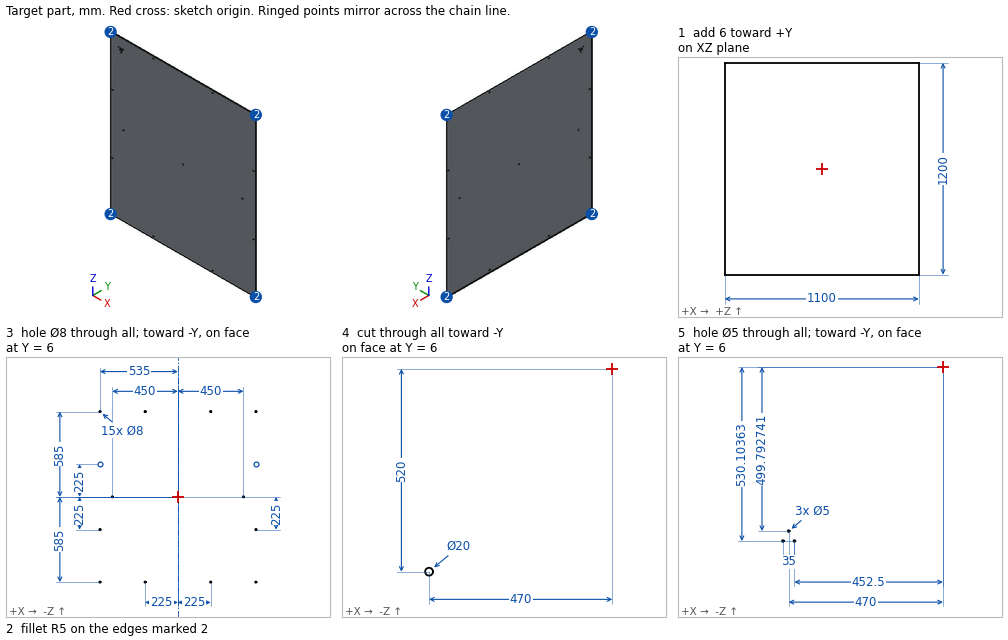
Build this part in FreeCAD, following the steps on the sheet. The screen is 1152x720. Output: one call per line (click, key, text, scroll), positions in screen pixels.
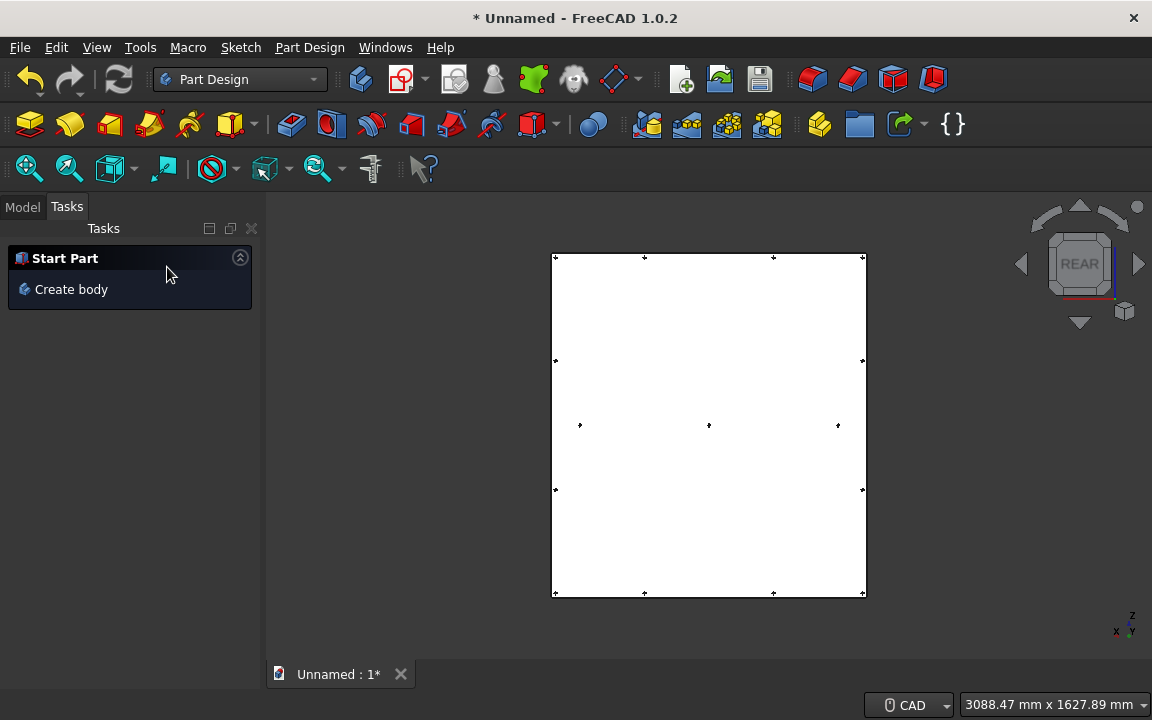
click(709, 523)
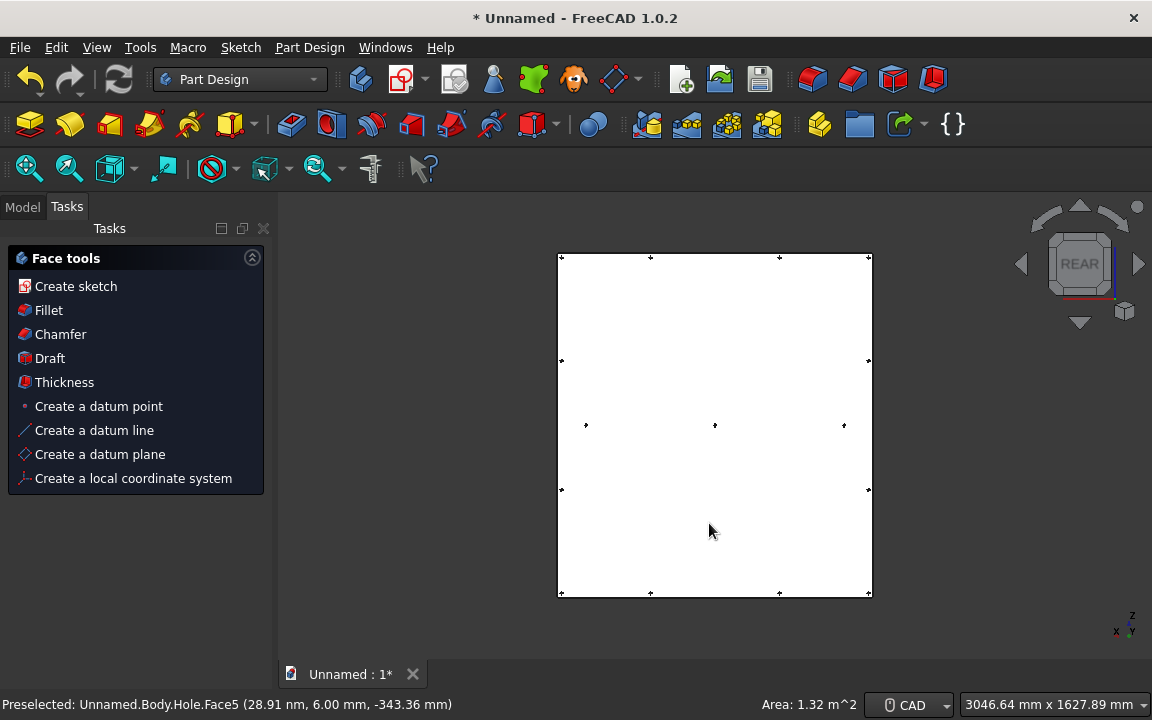
click(402, 80)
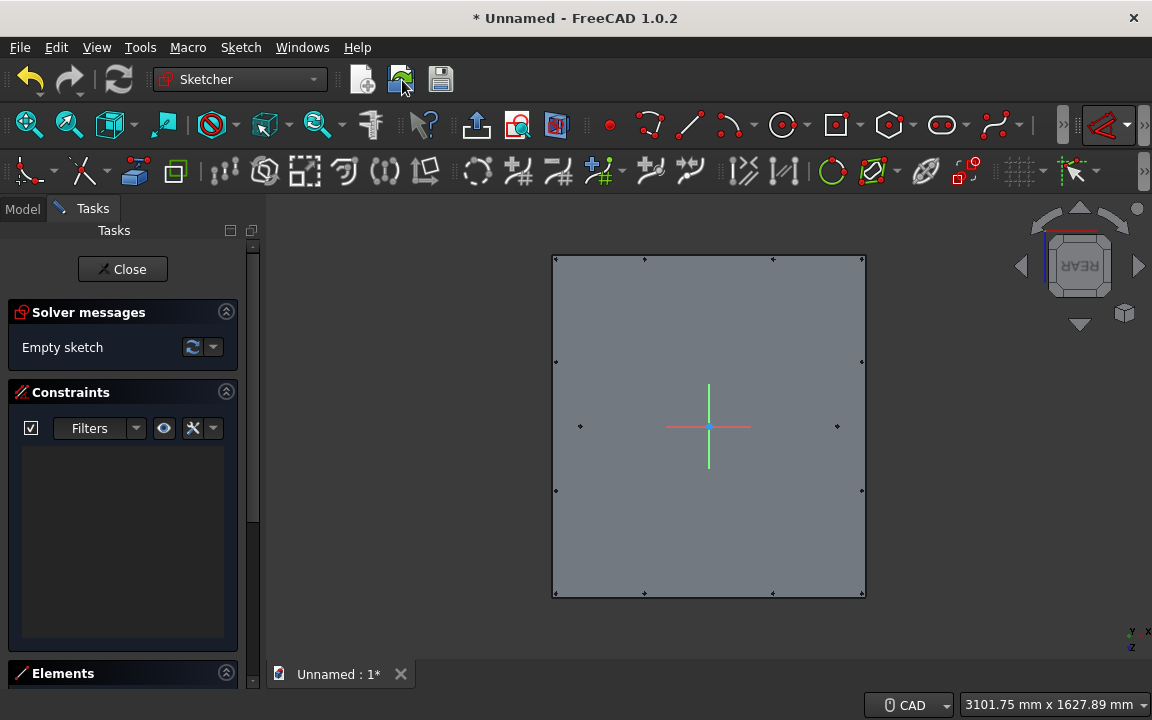
scroll(571, 583, up, 15)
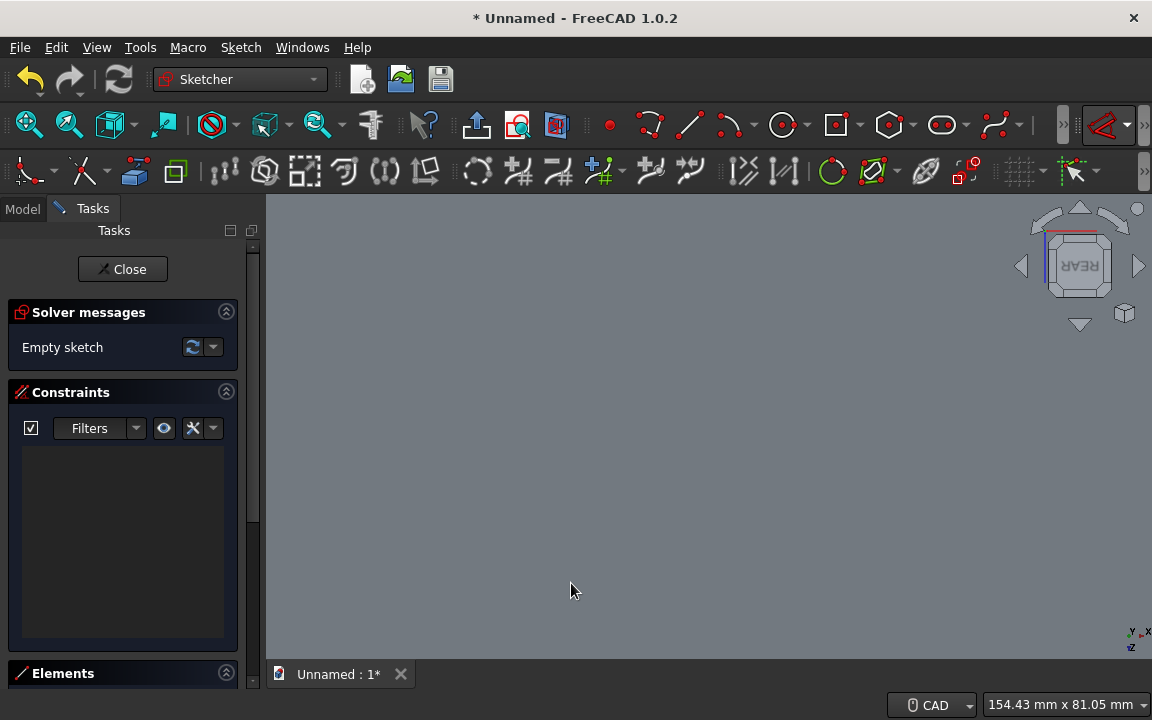
scroll(639, 396, up, 5)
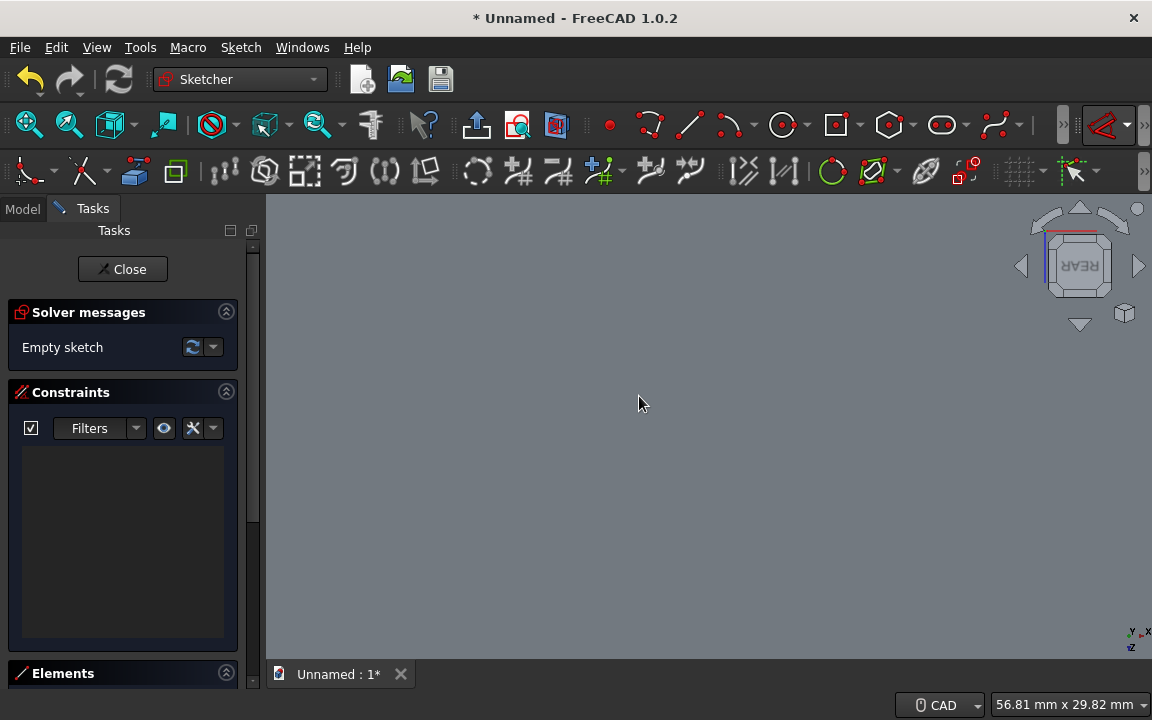
click(784, 126)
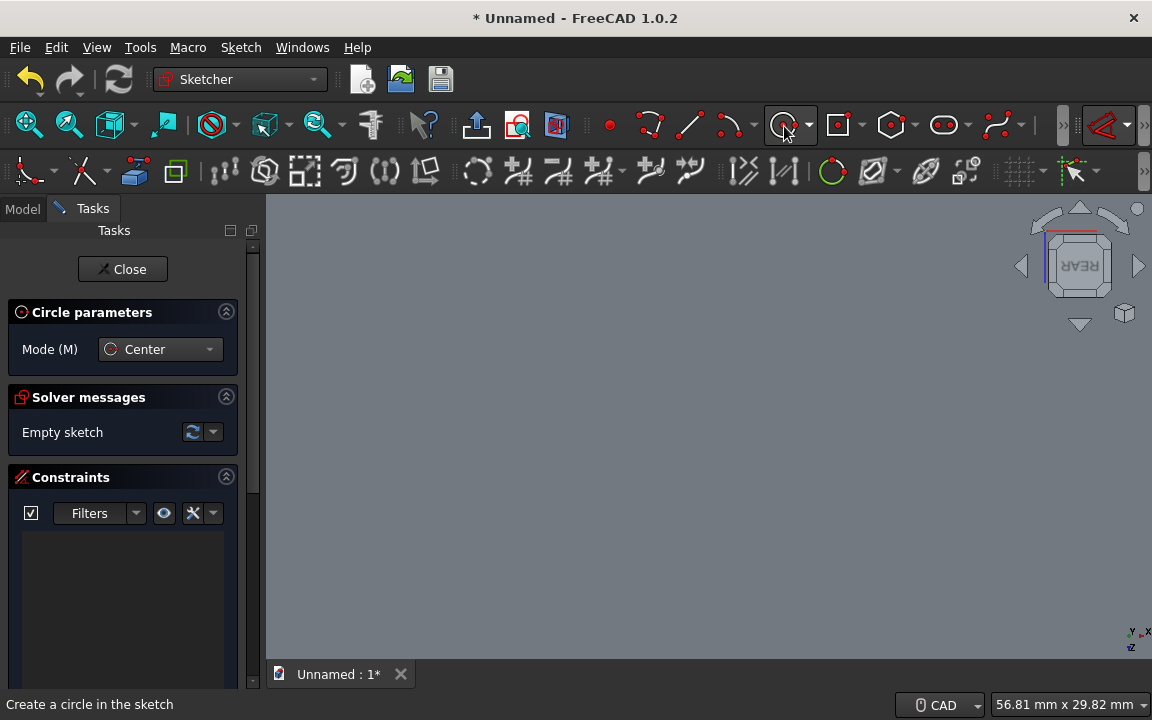
click(640, 425)
move(750, 315)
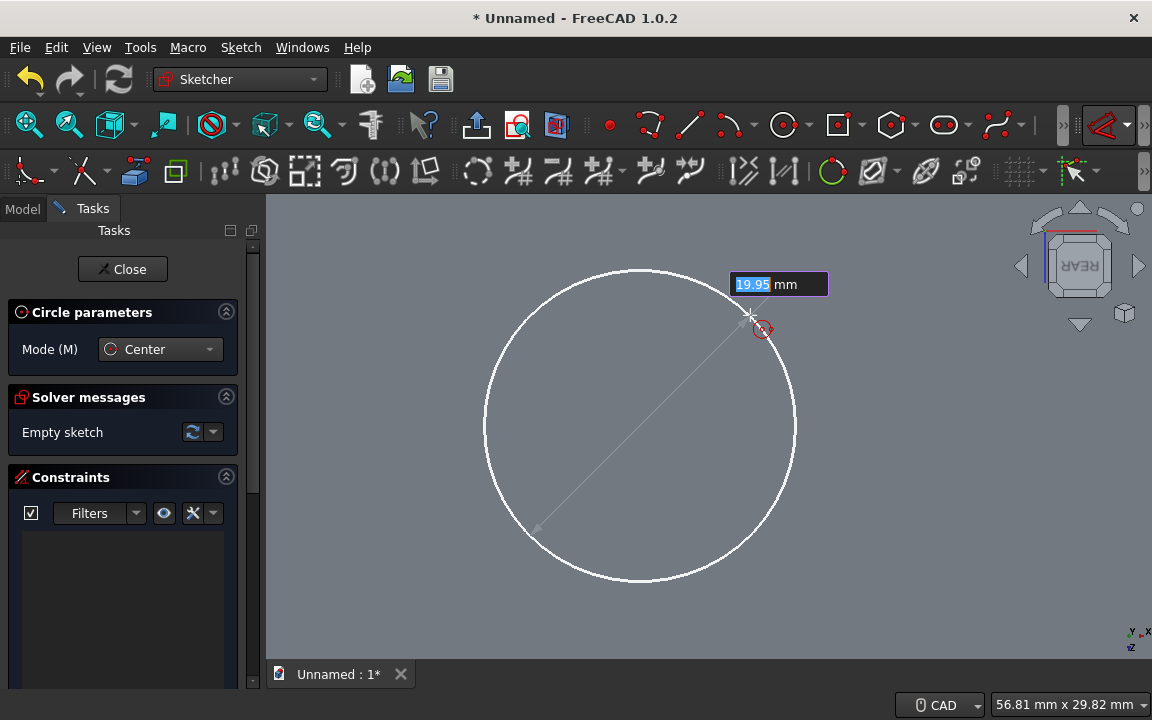
text(20)
key(Return)
key(Escape)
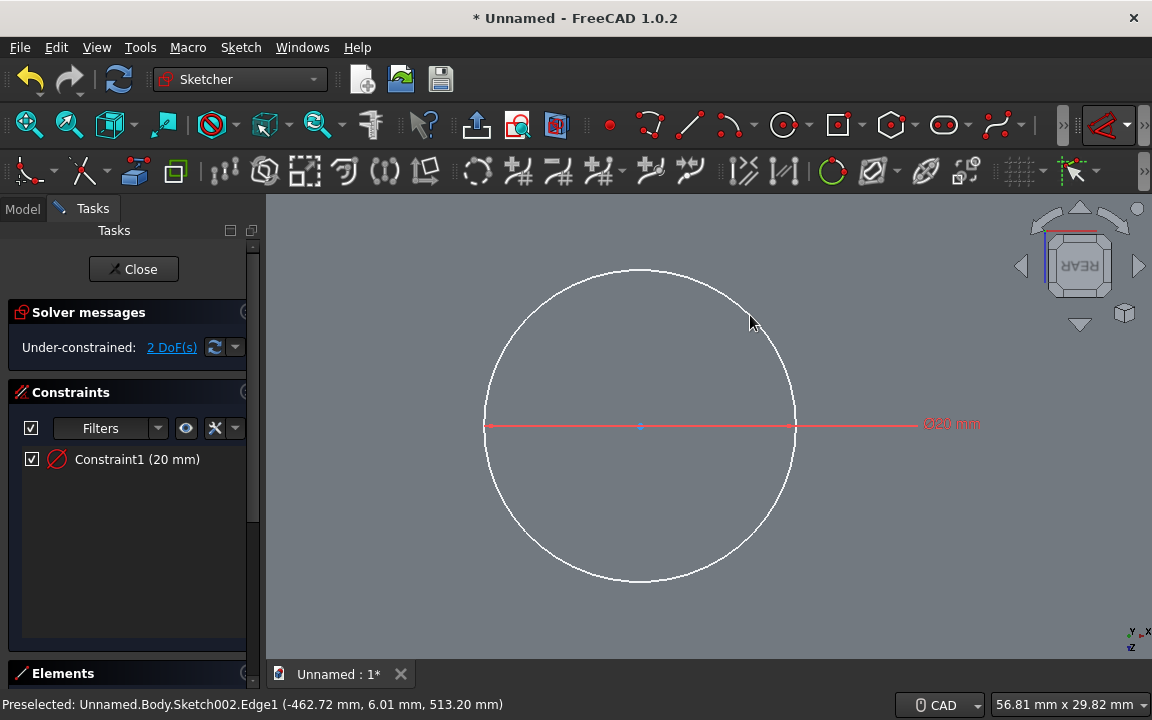
click(640, 426)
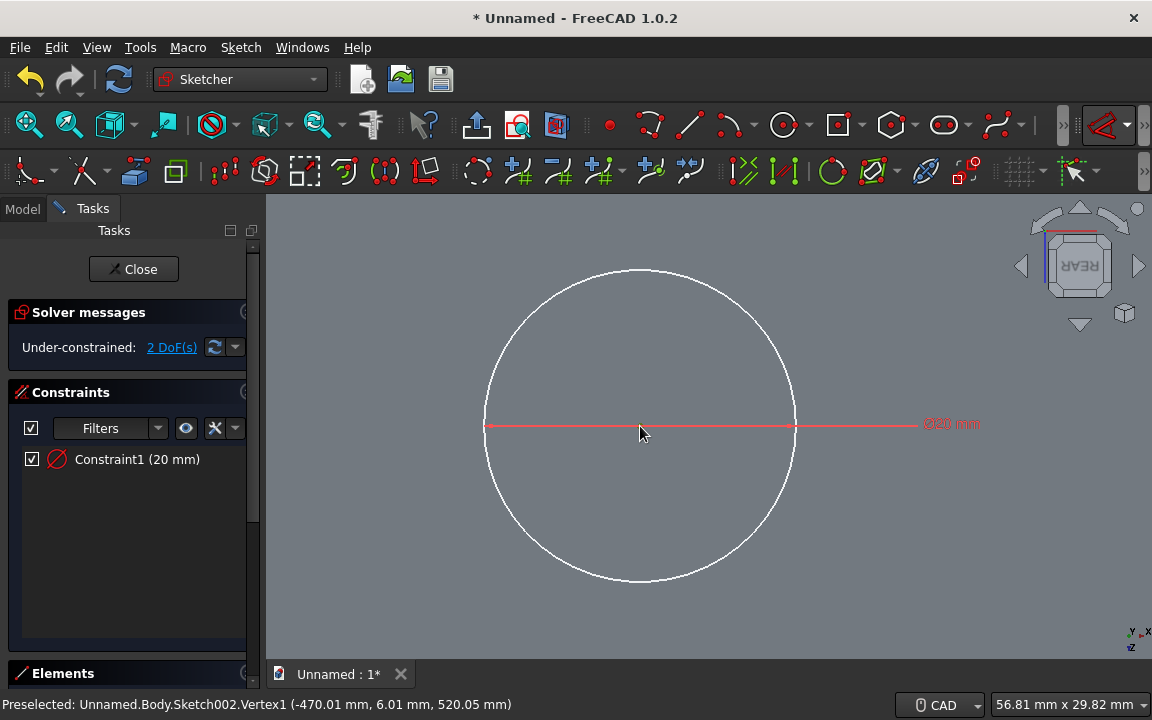
key(l)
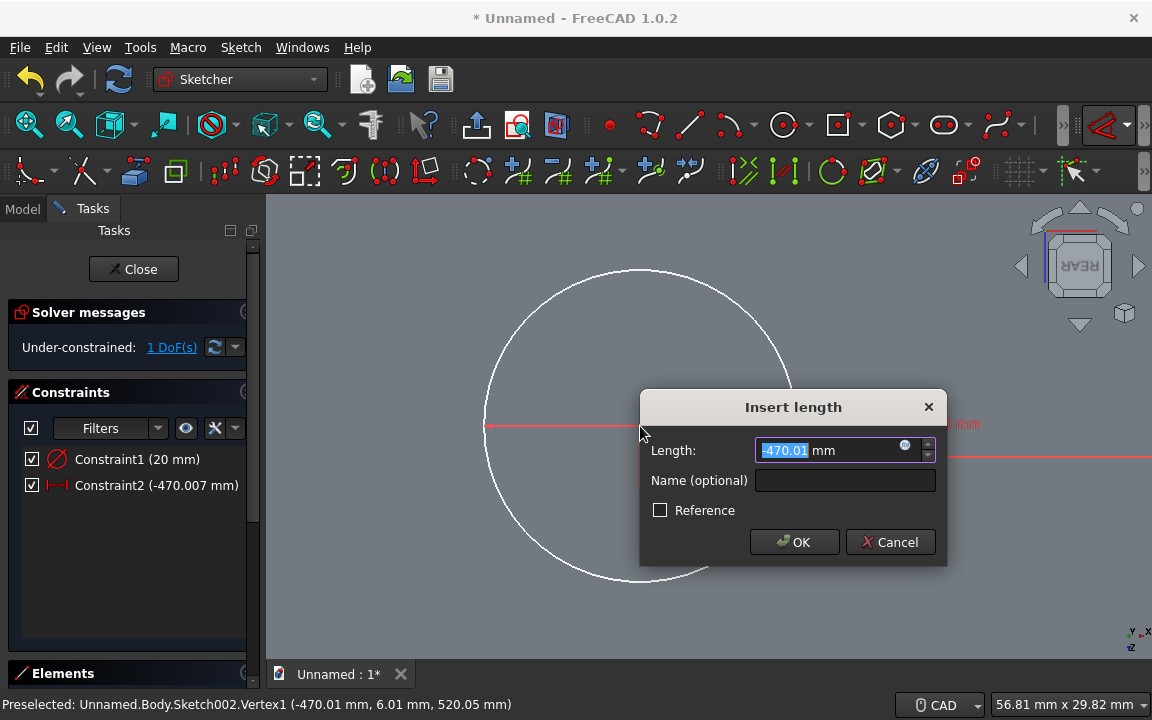
text(-470)
key(Return)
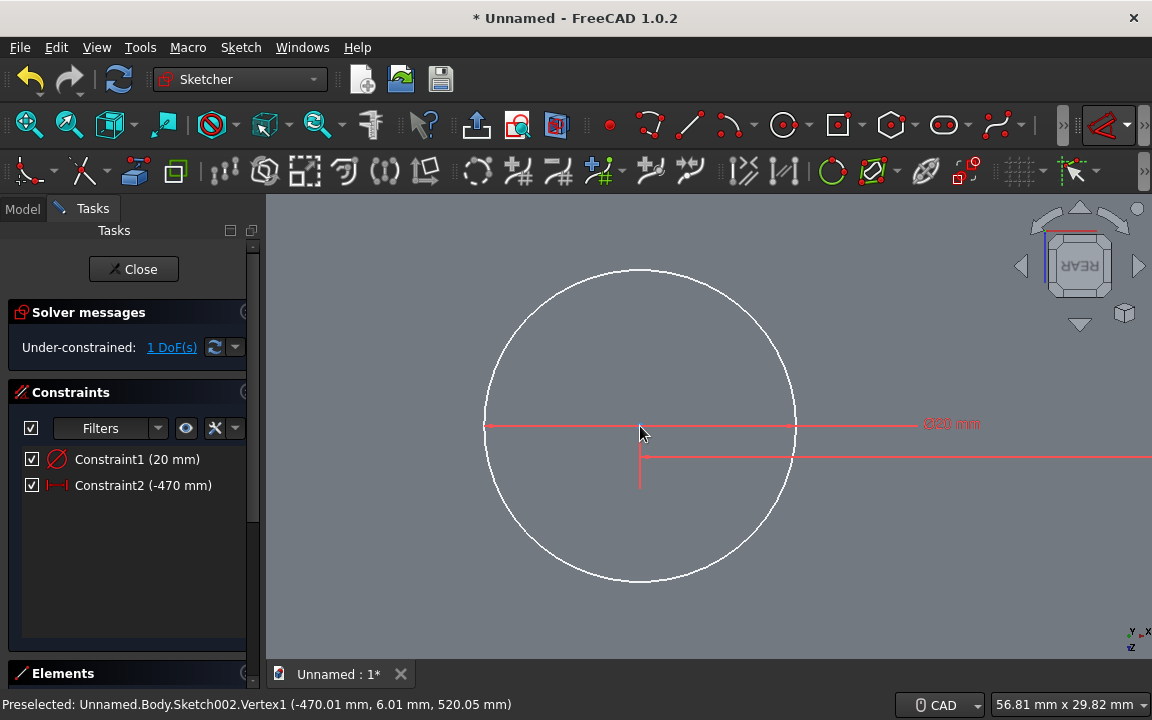
click(640, 426)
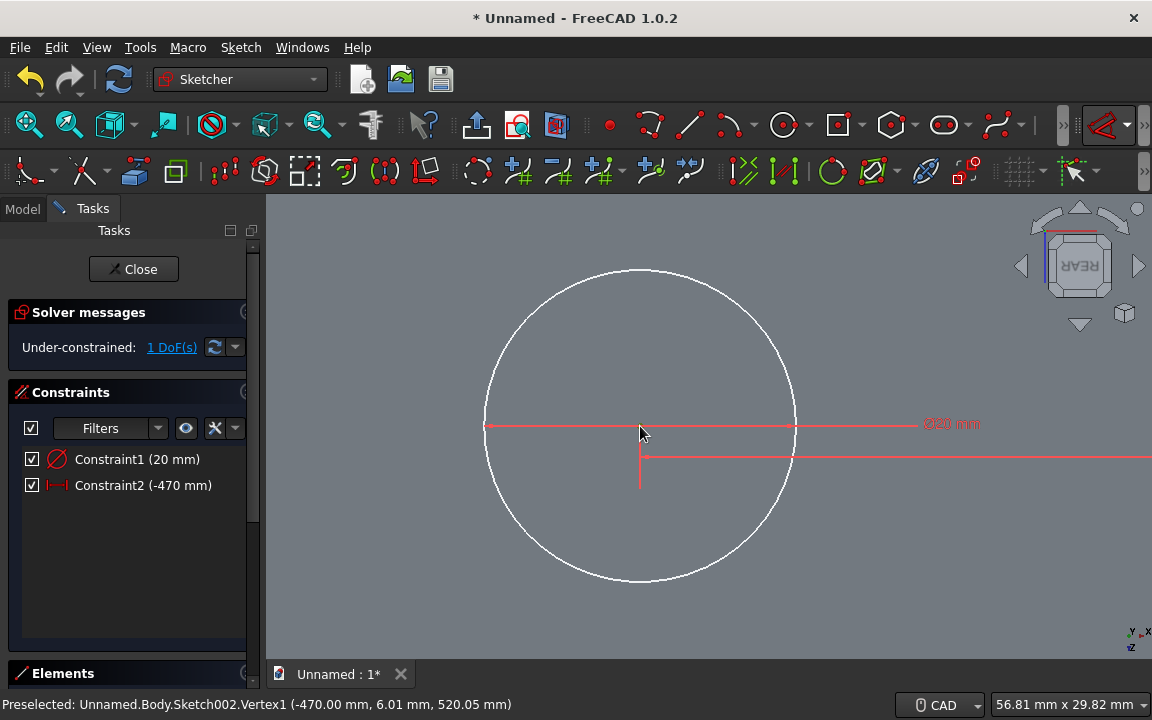
click(1130, 126)